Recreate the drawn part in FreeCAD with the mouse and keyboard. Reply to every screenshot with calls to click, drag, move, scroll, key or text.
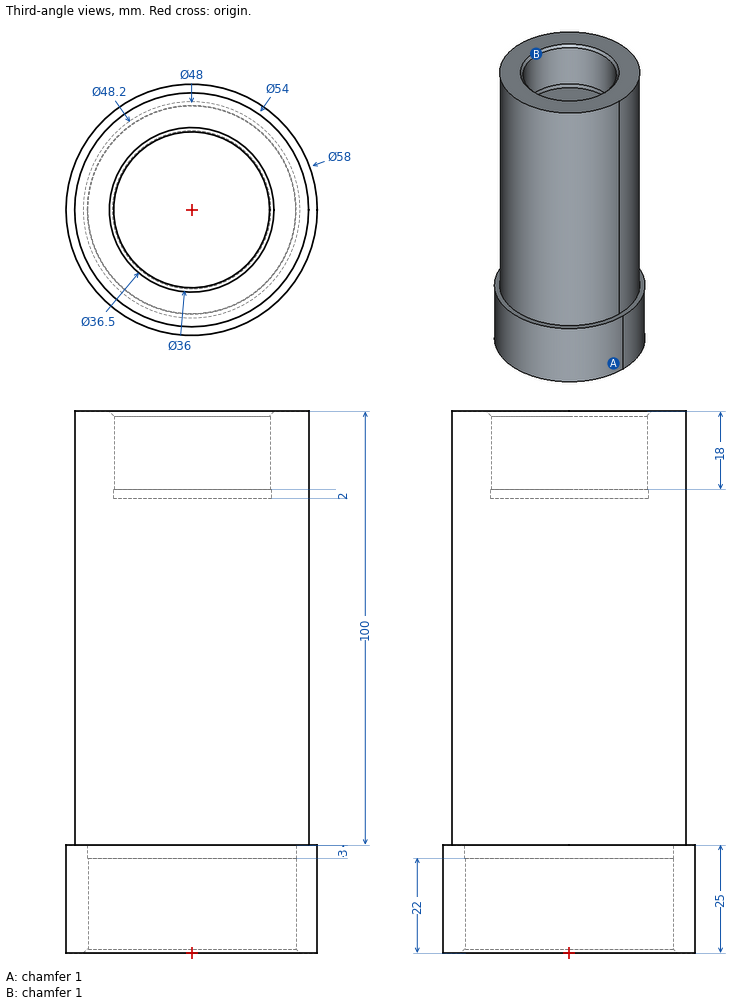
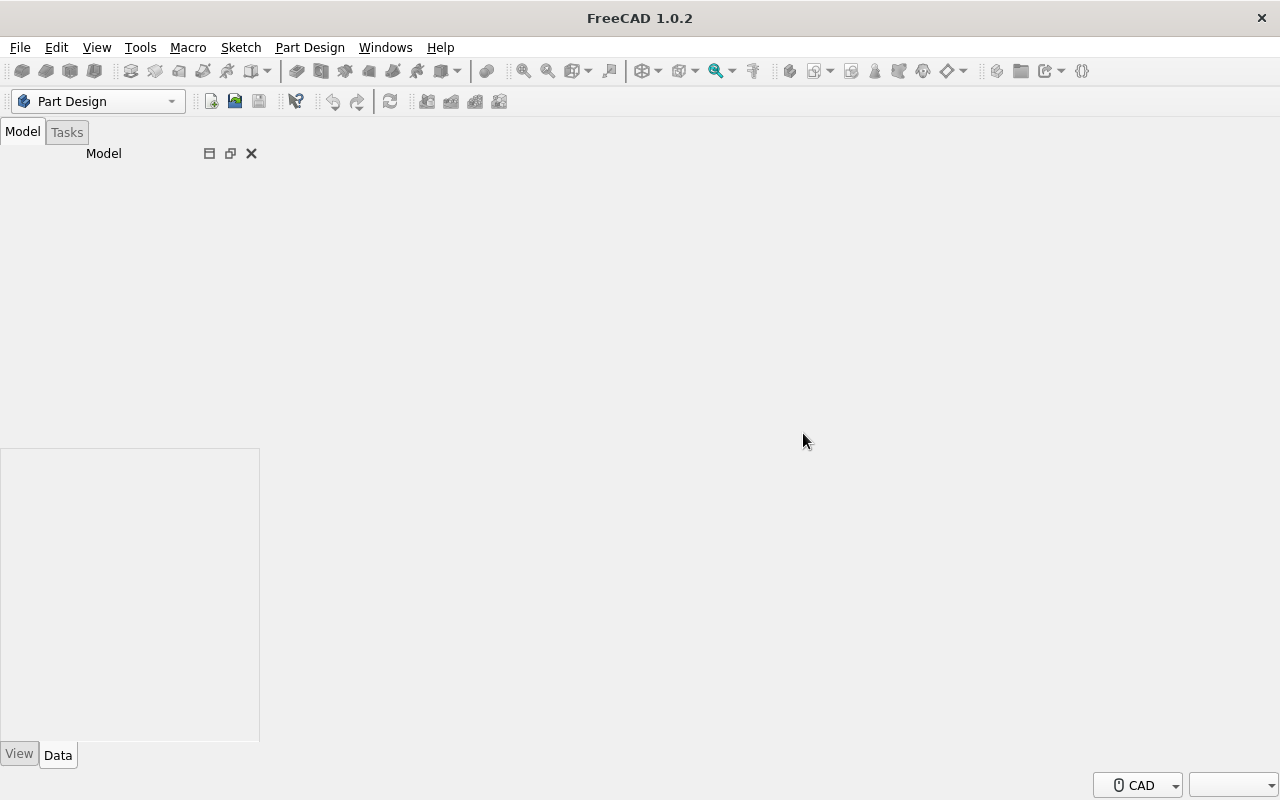
click(212, 102)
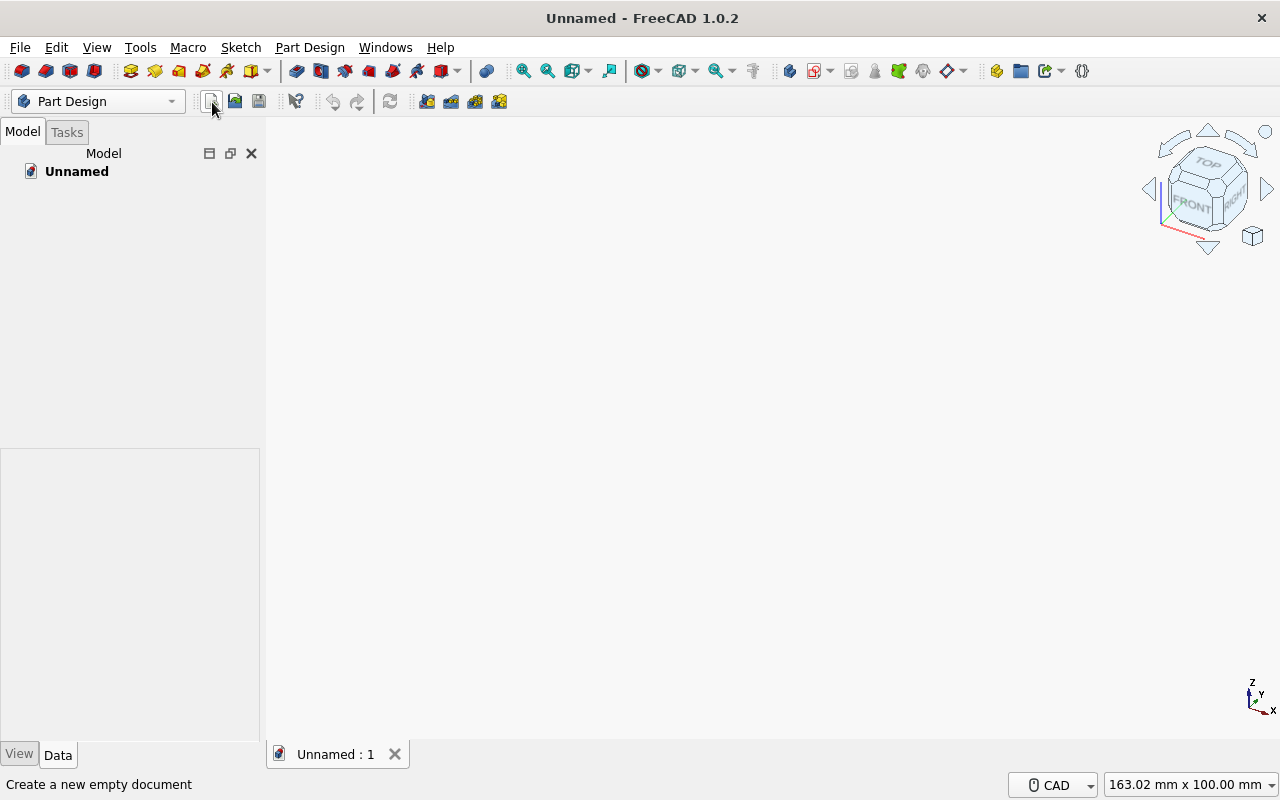
click(814, 72)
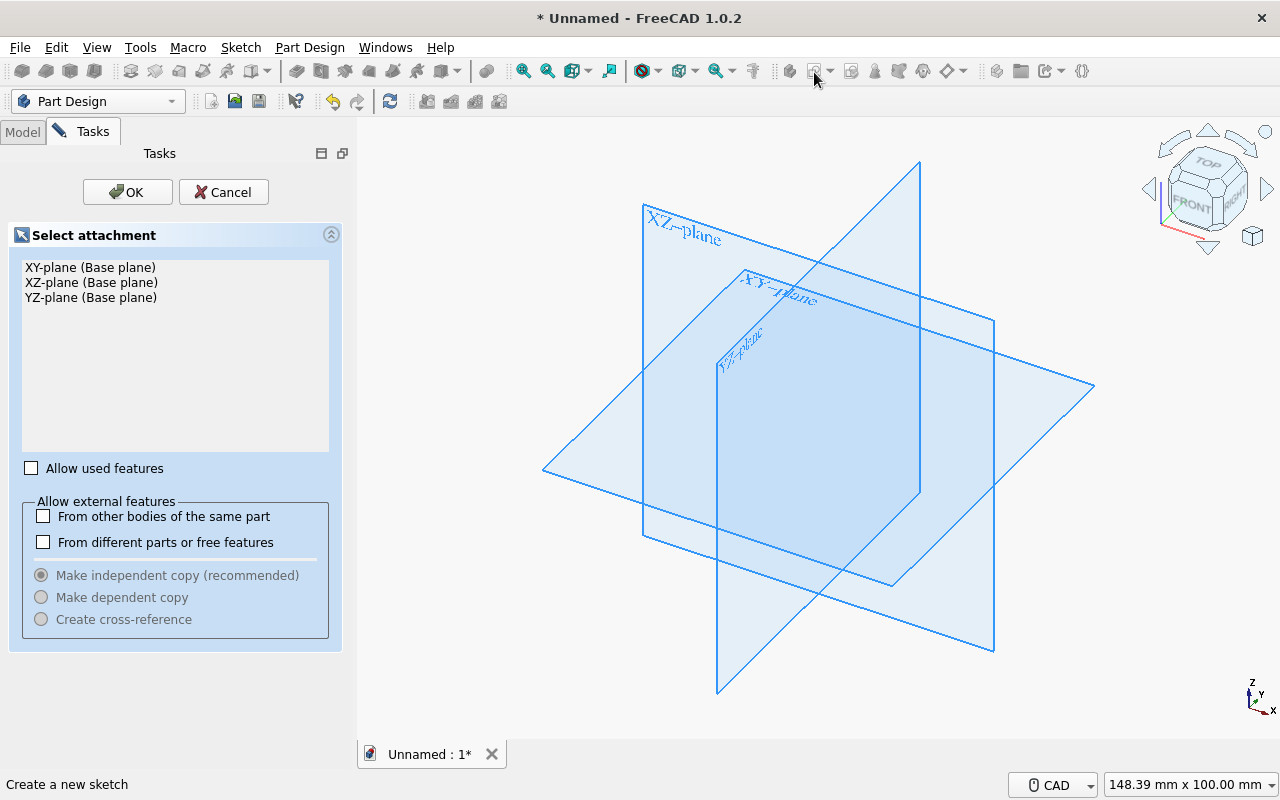
click(82, 268)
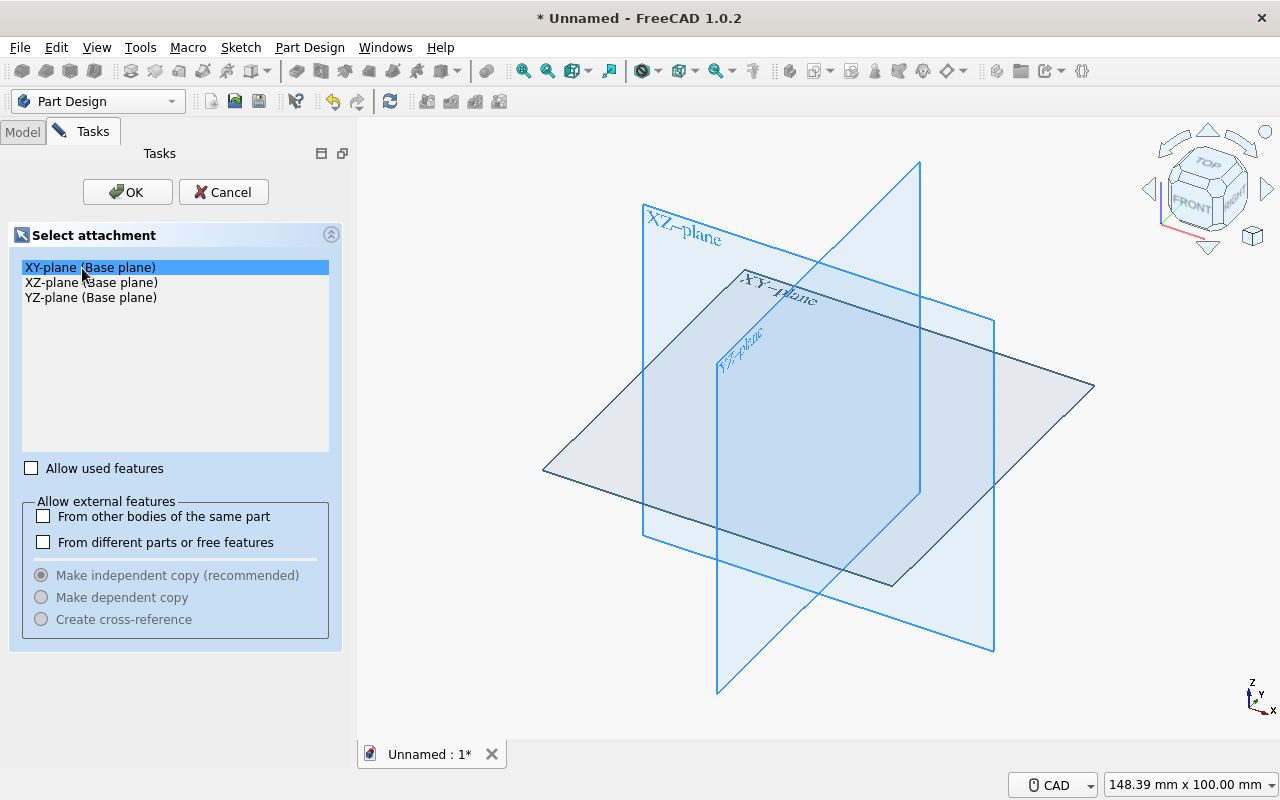
click(128, 192)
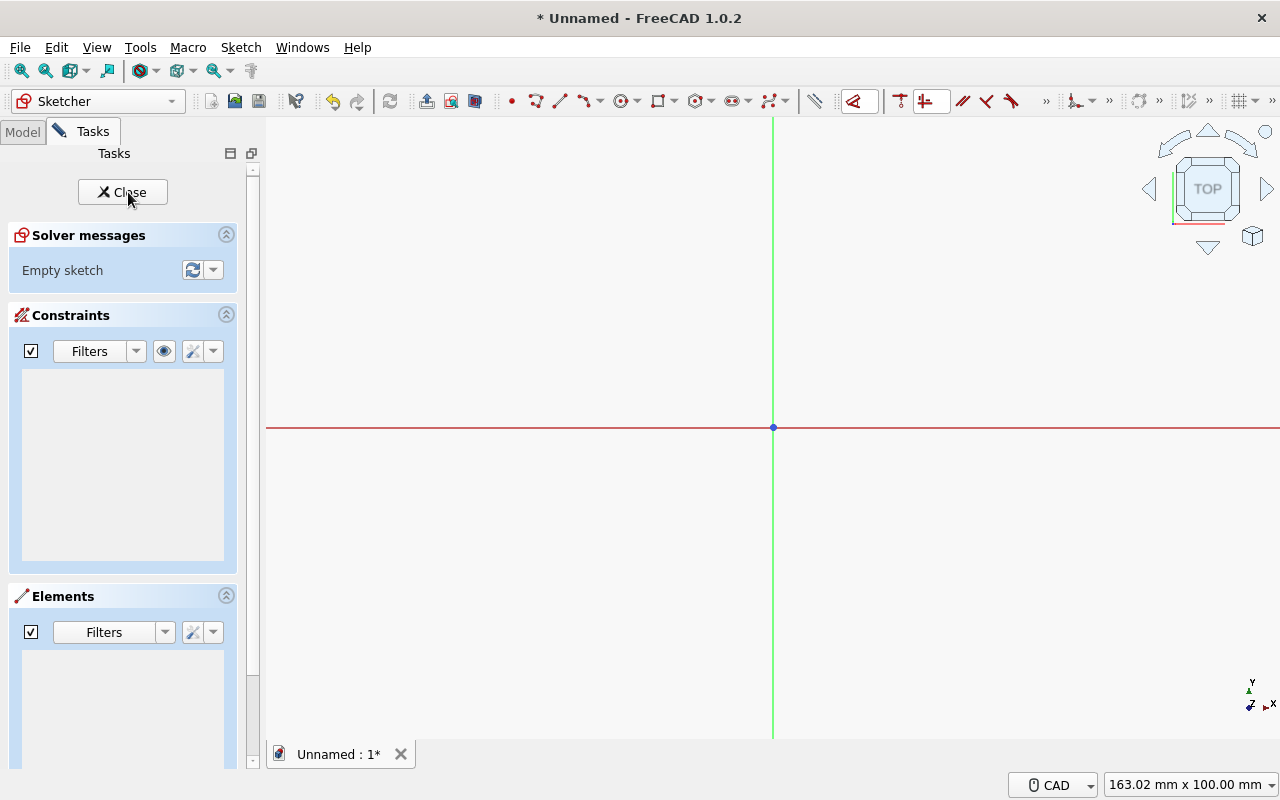
click(622, 102)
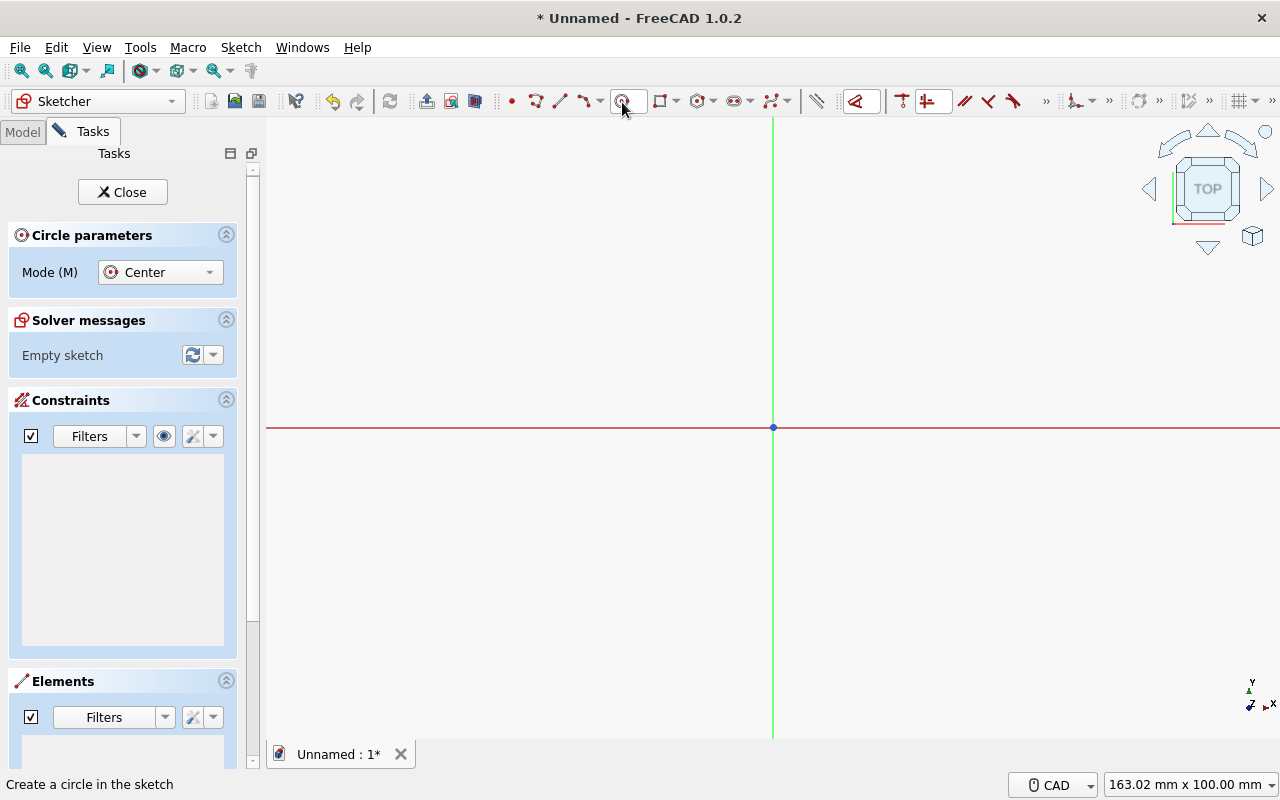
click(773, 428)
move(901, 300)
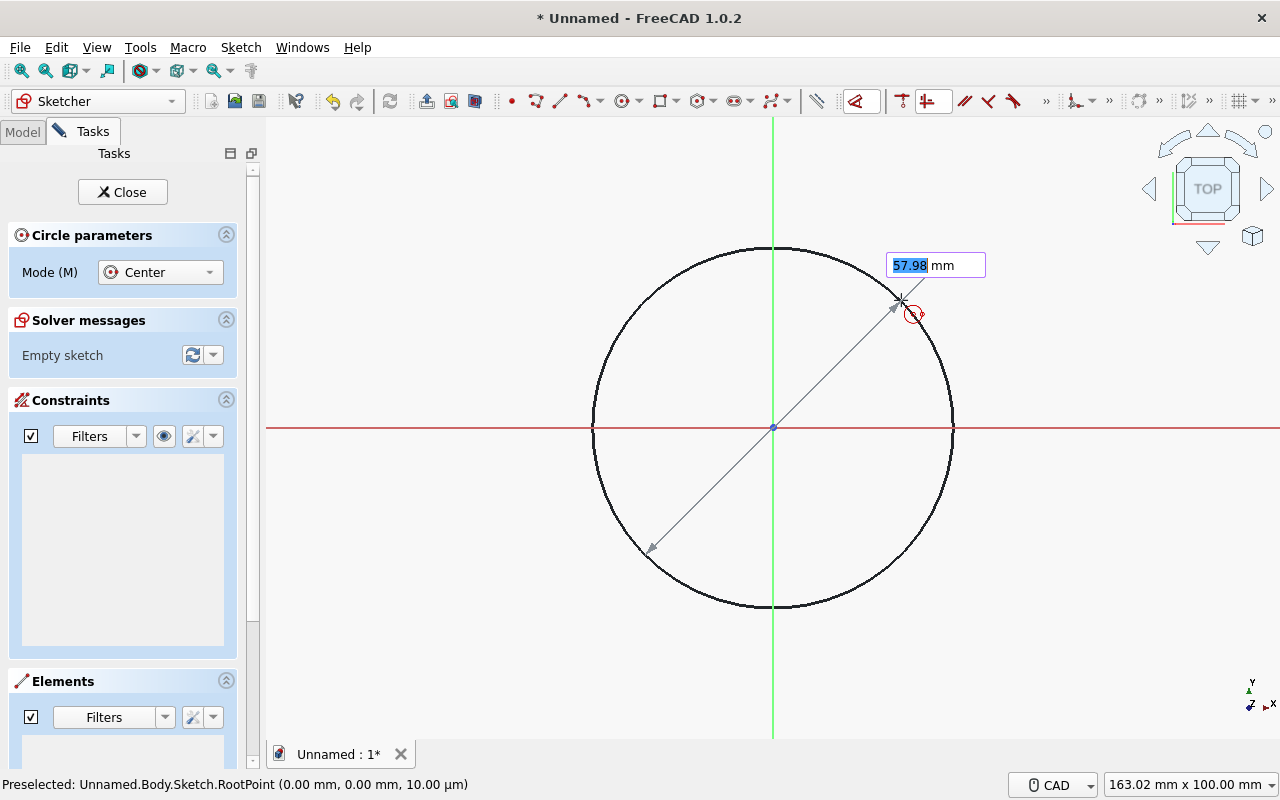
text(58)
key(Return)
key(Escape)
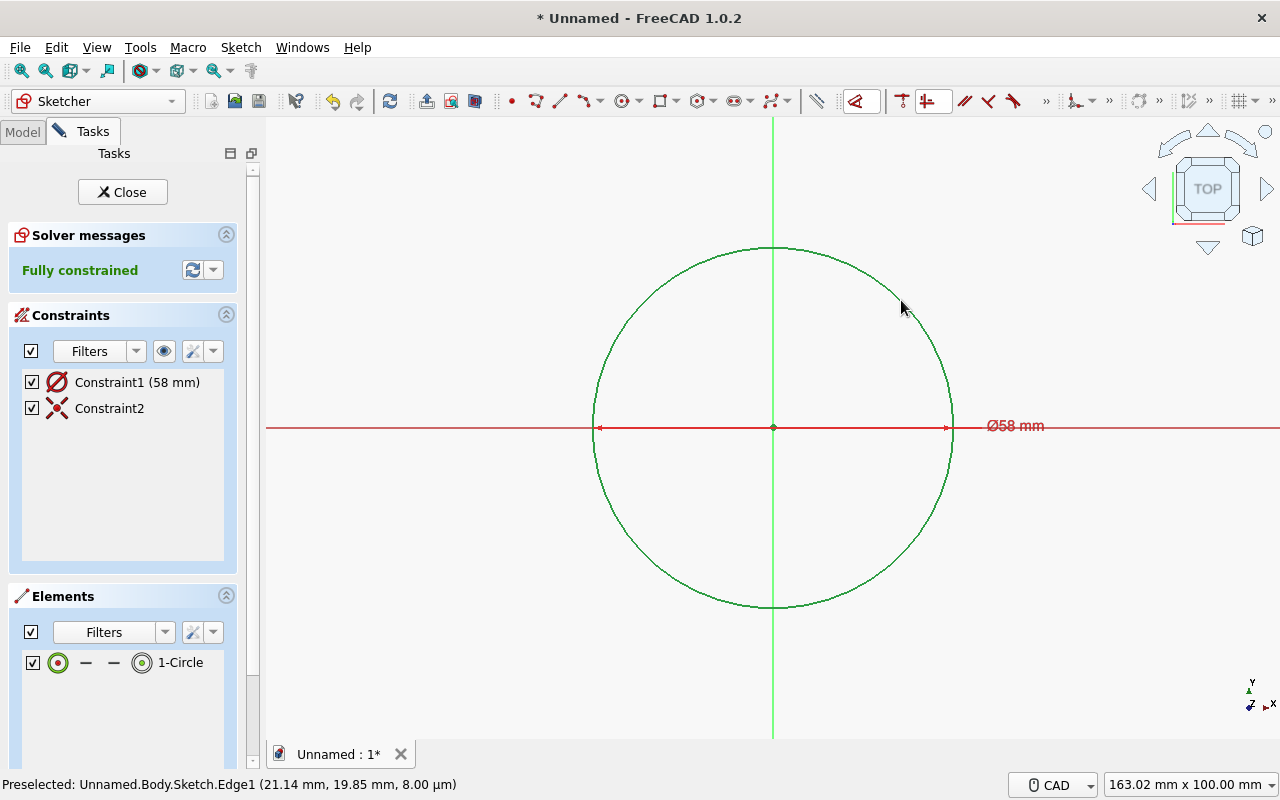
click(123, 192)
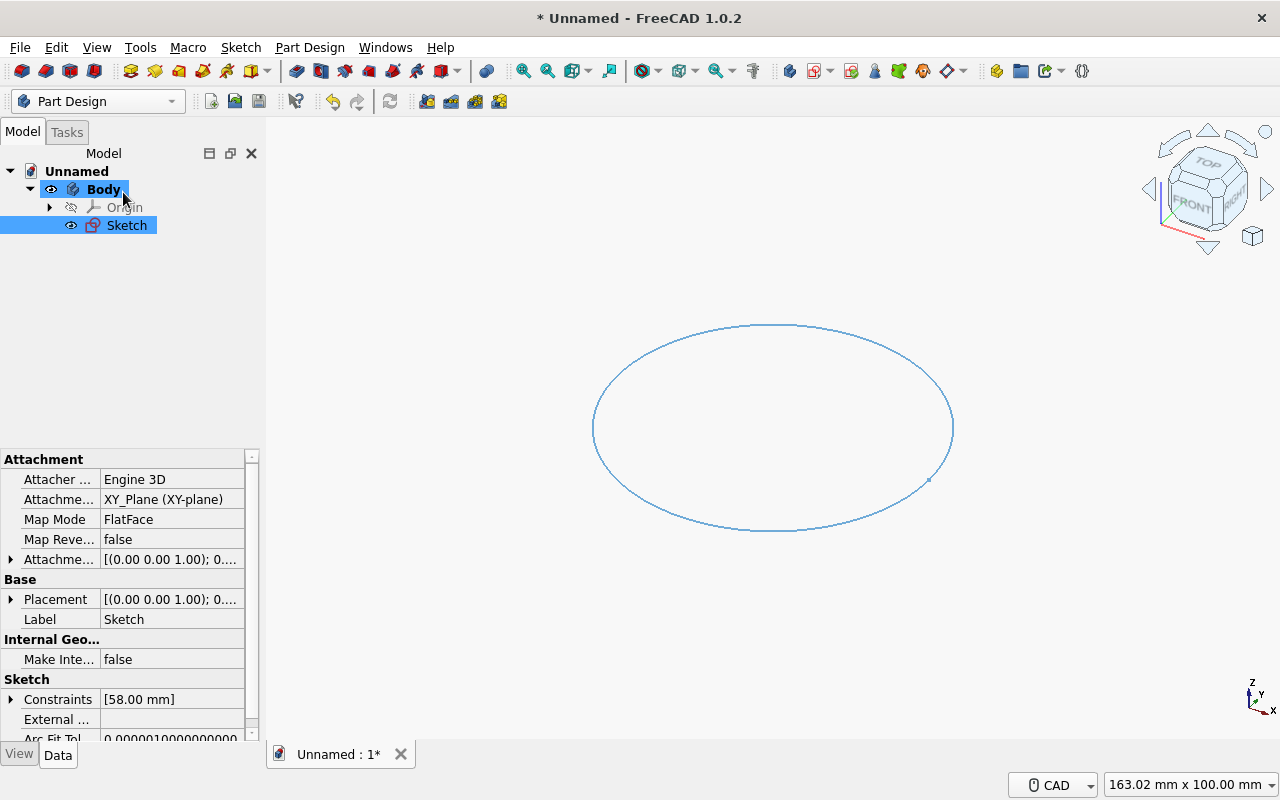
click(132, 72)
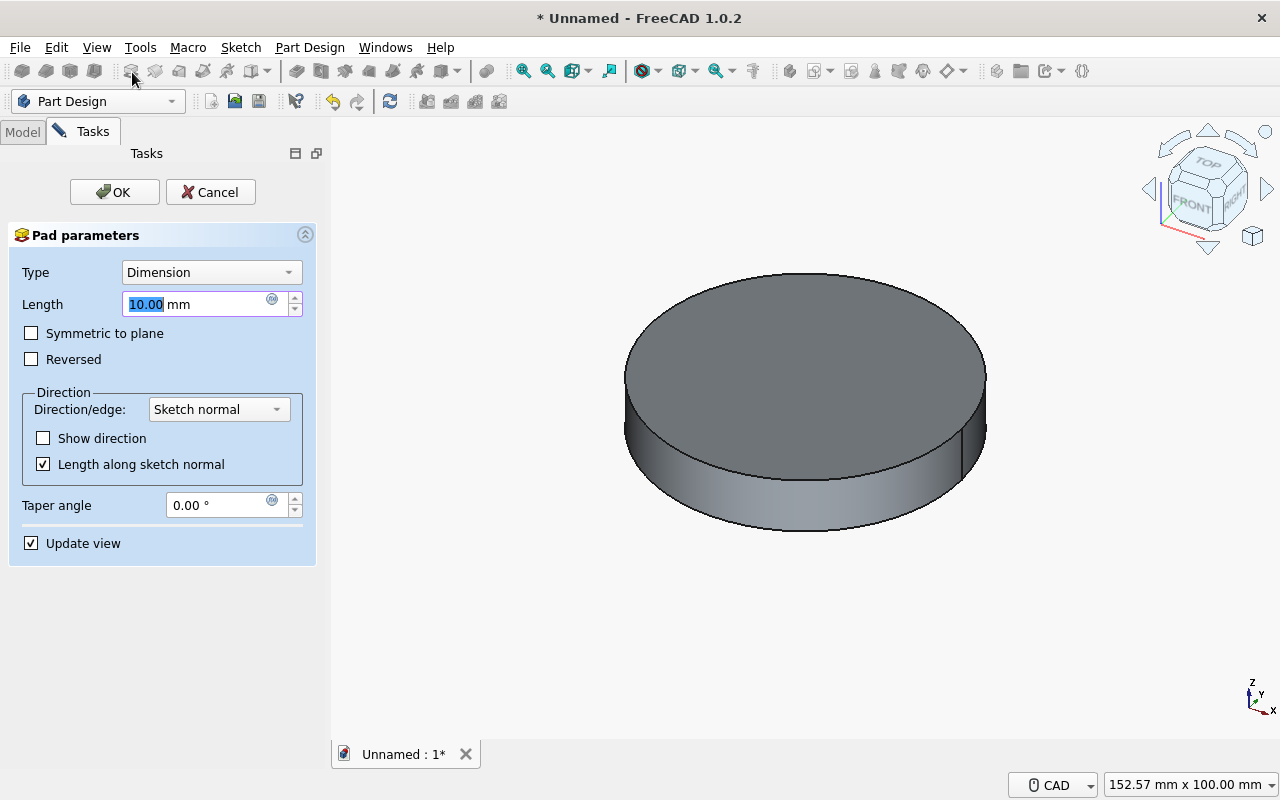
text(25)
key(Tab)